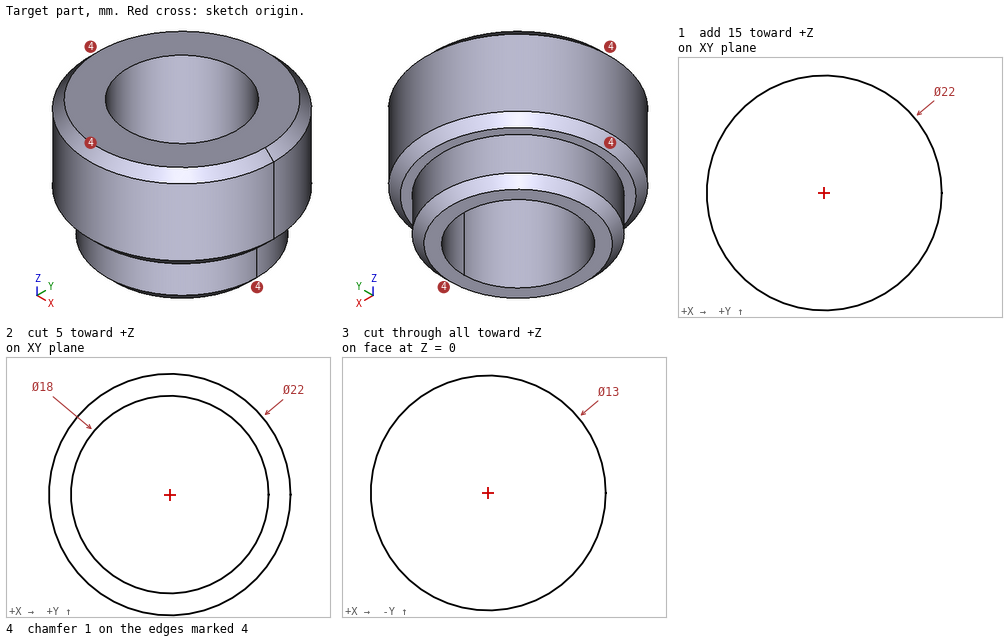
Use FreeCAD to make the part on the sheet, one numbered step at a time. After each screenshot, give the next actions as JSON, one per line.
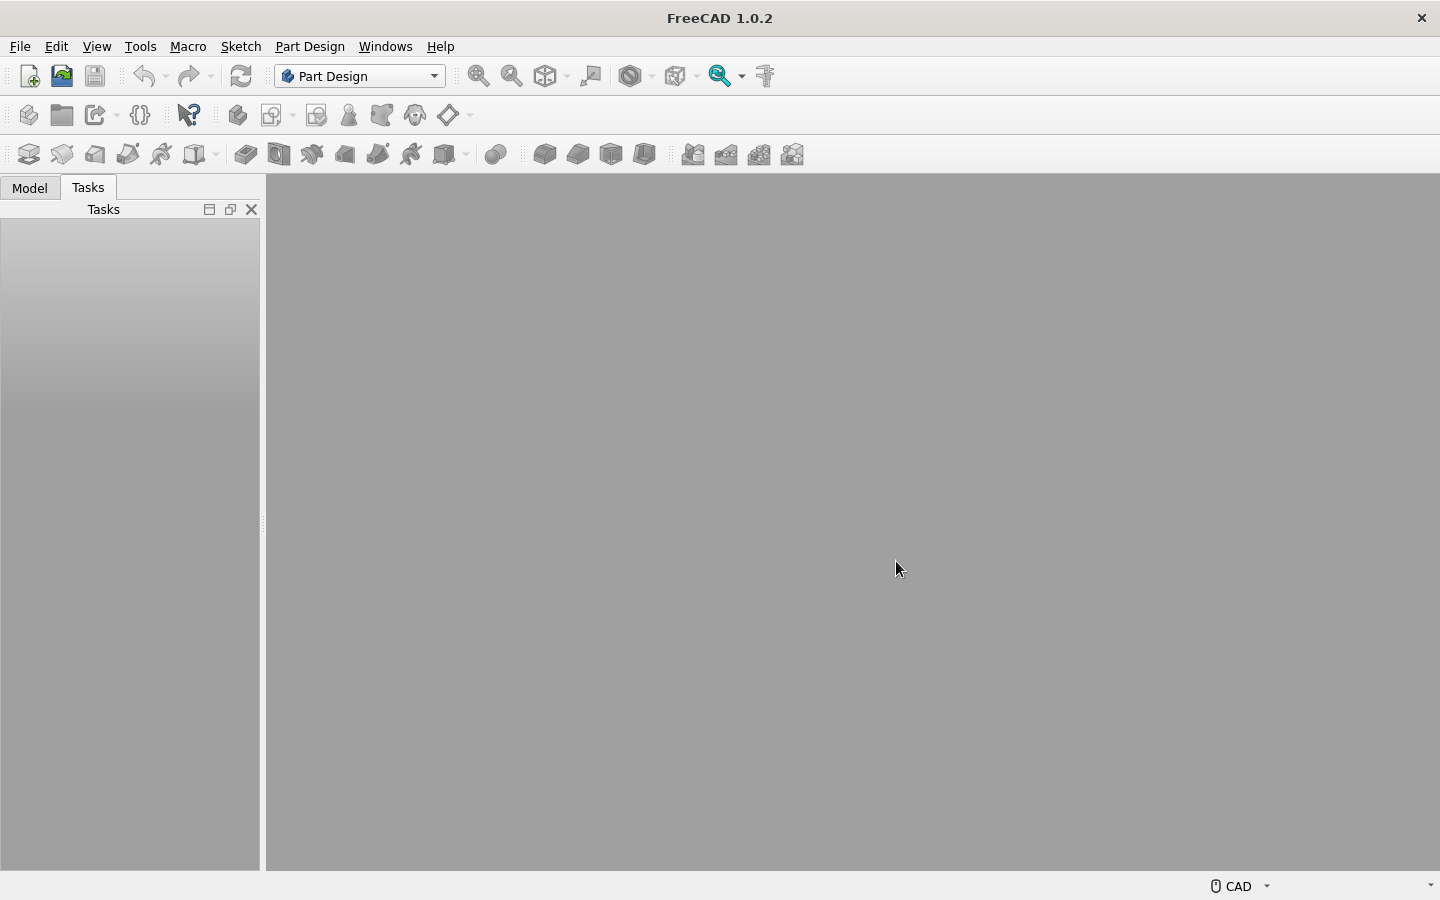
{"action": "key", "text": "ctrl+n"}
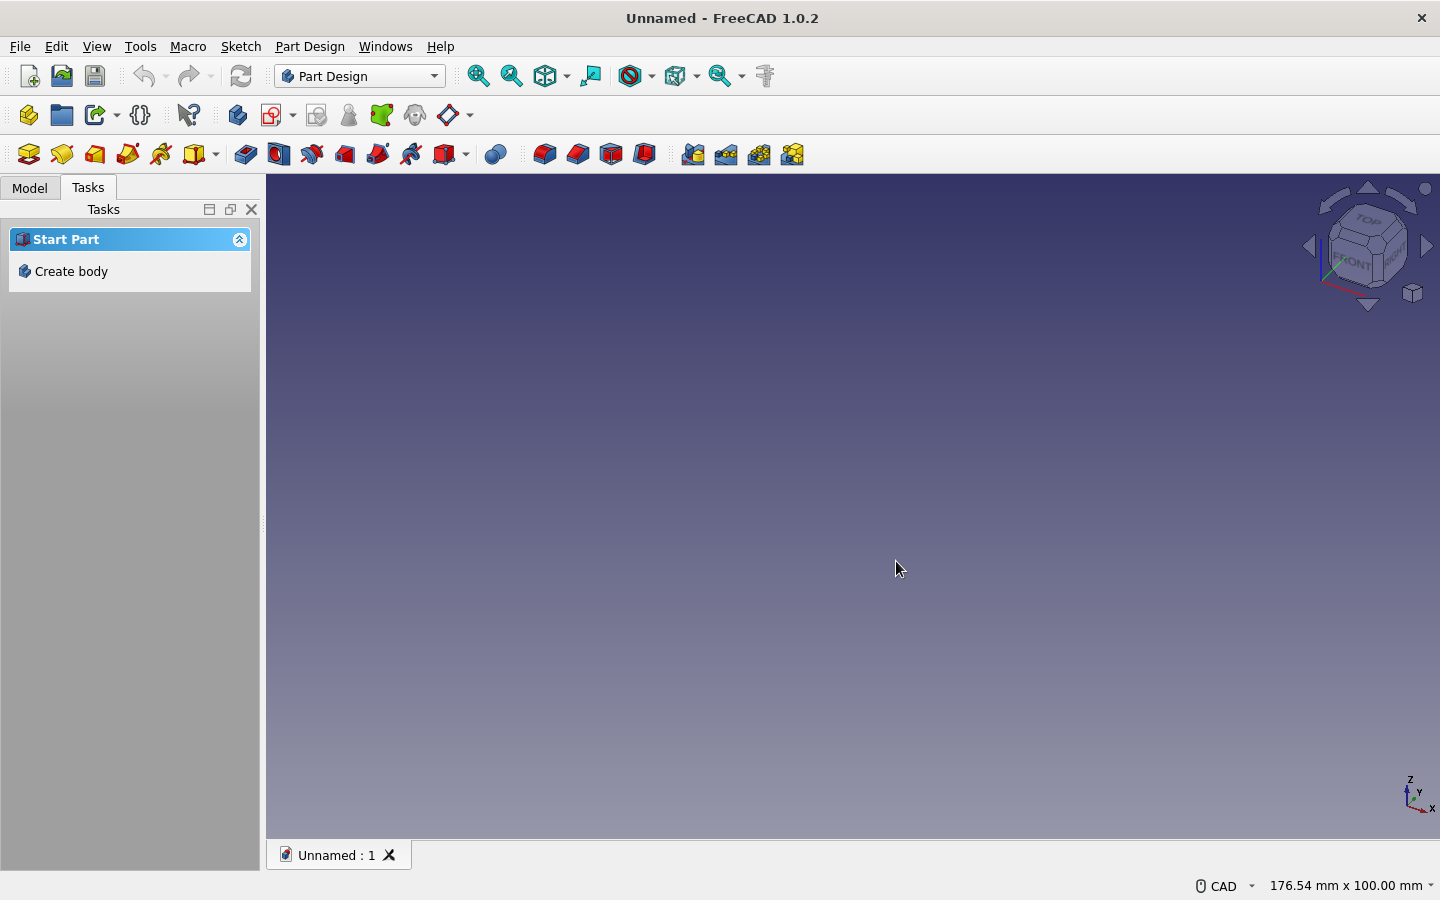
{"action": "left_click", "coordinate": [270, 116]}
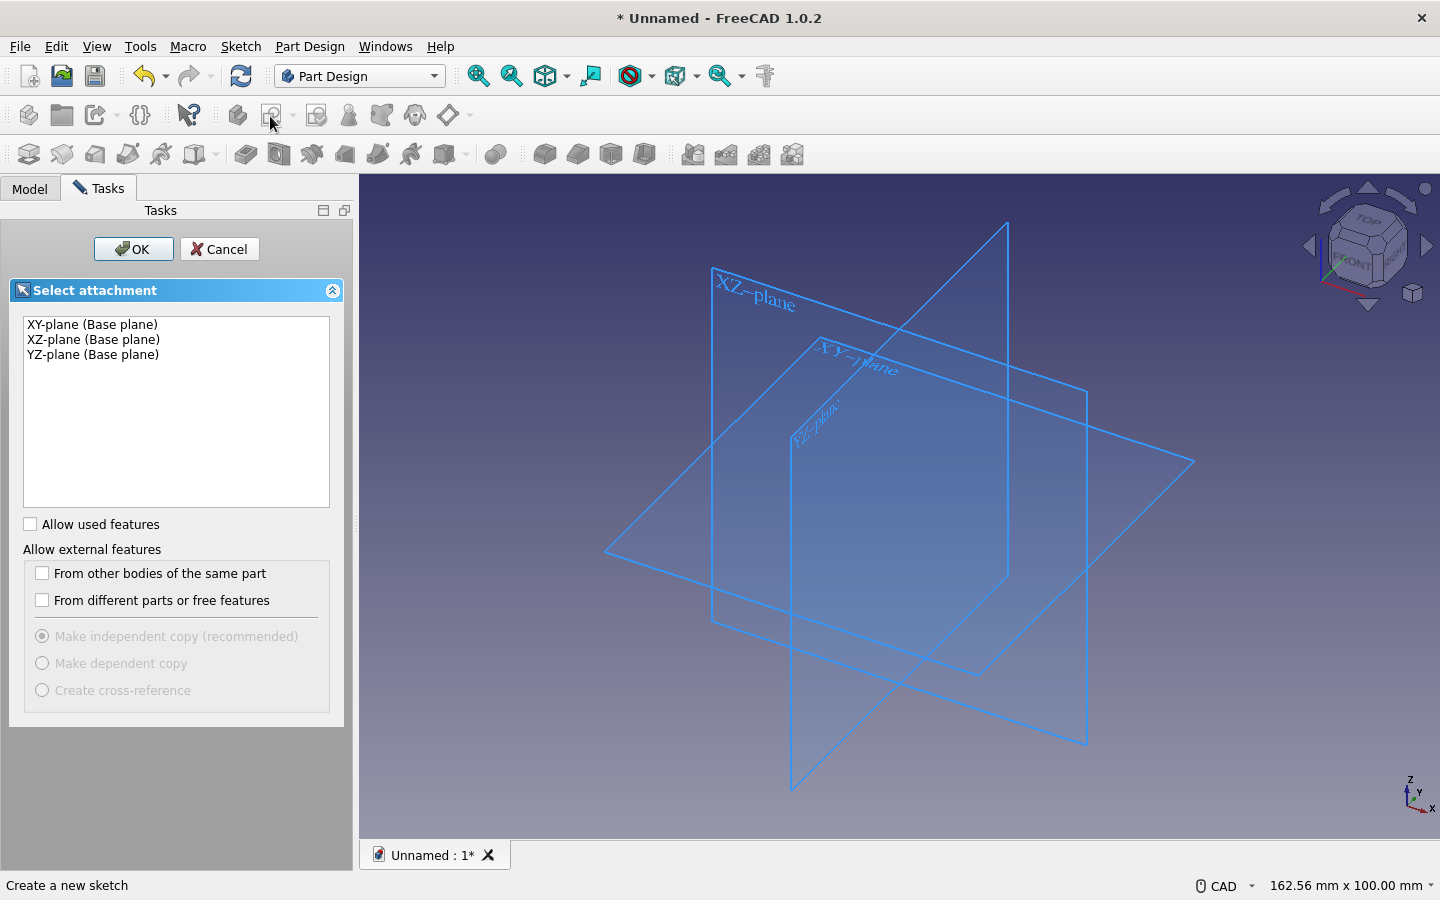
{"action": "left_click", "coordinate": [84, 324]}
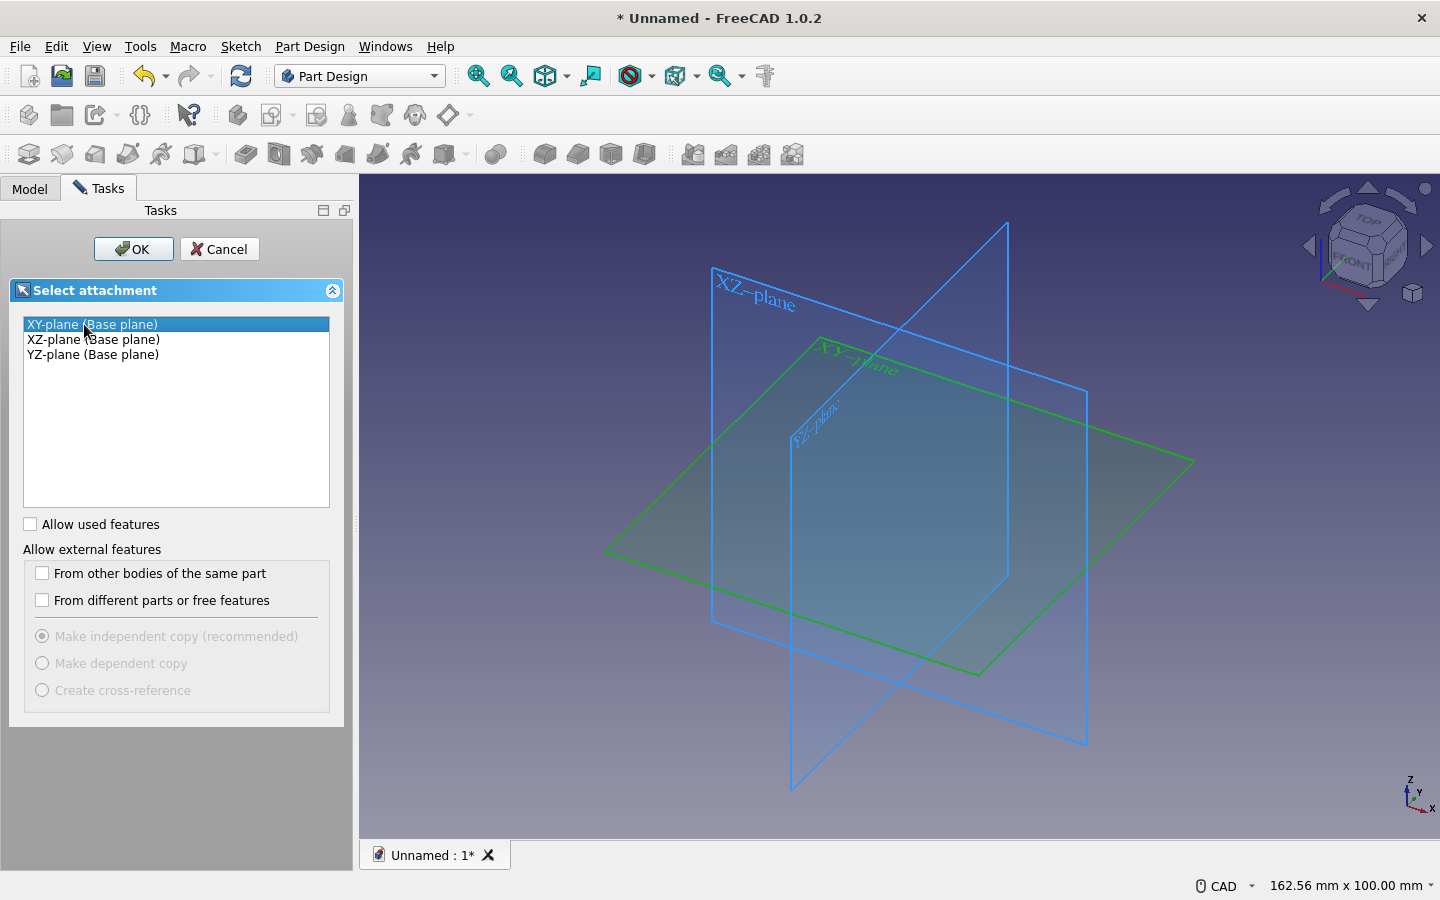
{"action": "left_click", "coordinate": [134, 249]}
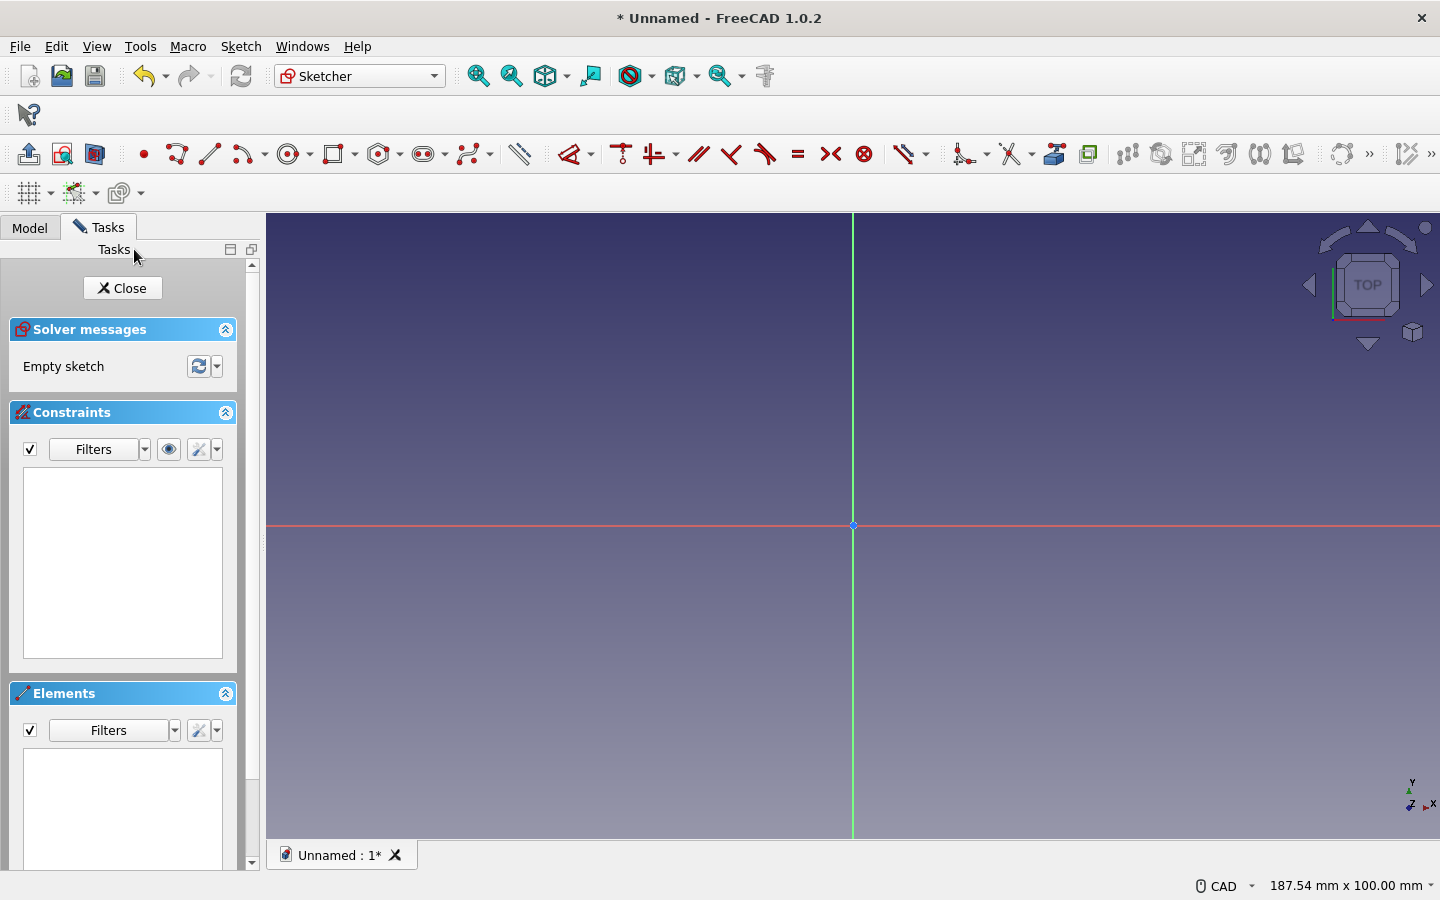
{"action": "scroll", "coordinate": [893, 526], "scroll_direction": "up", "scroll_amount": 5}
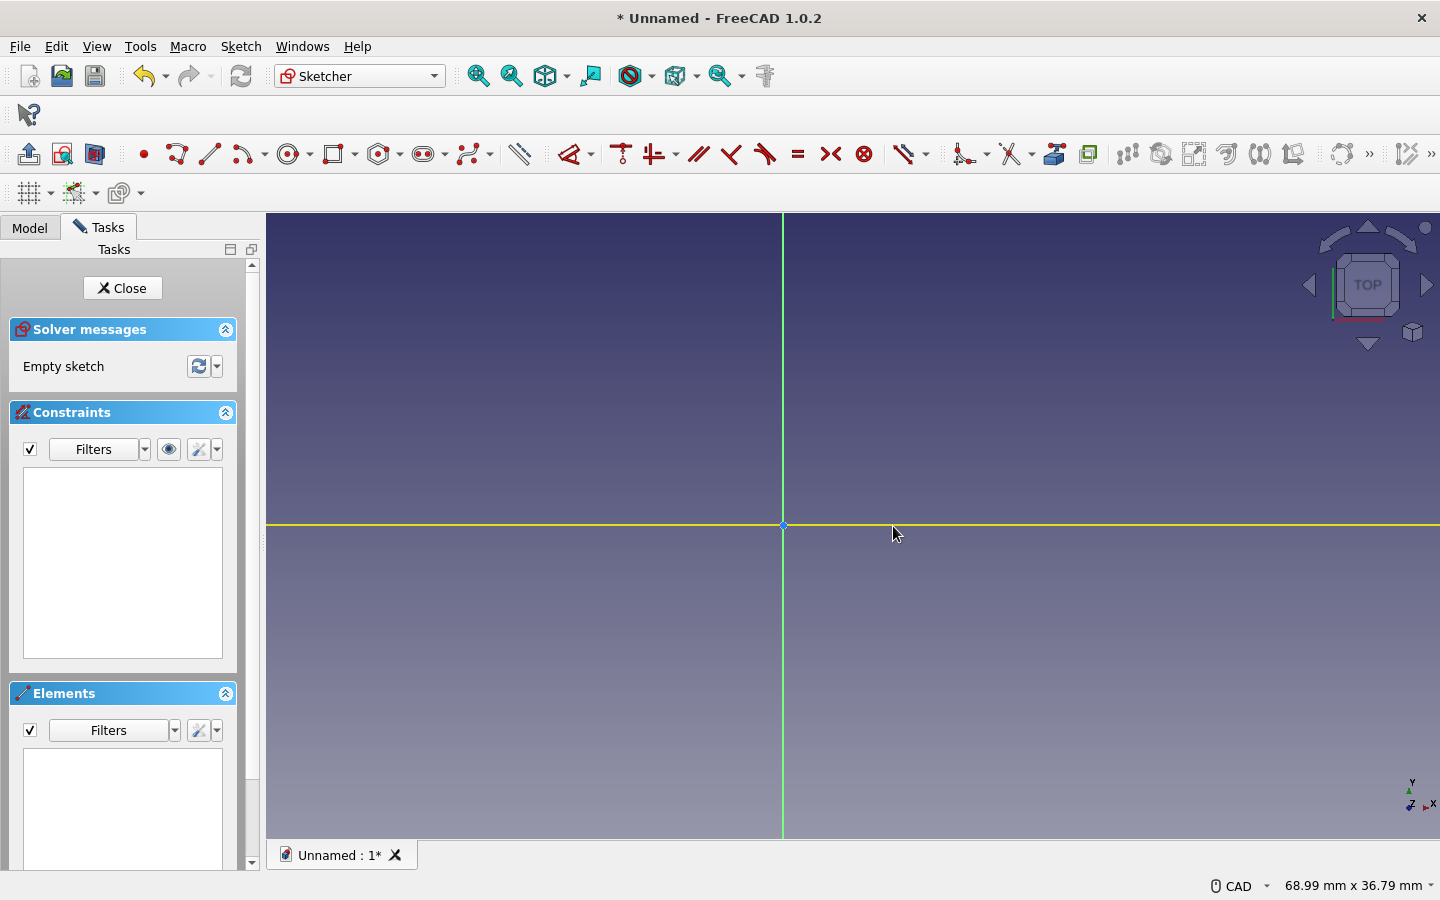
{"action": "left_click", "coordinate": [288, 154]}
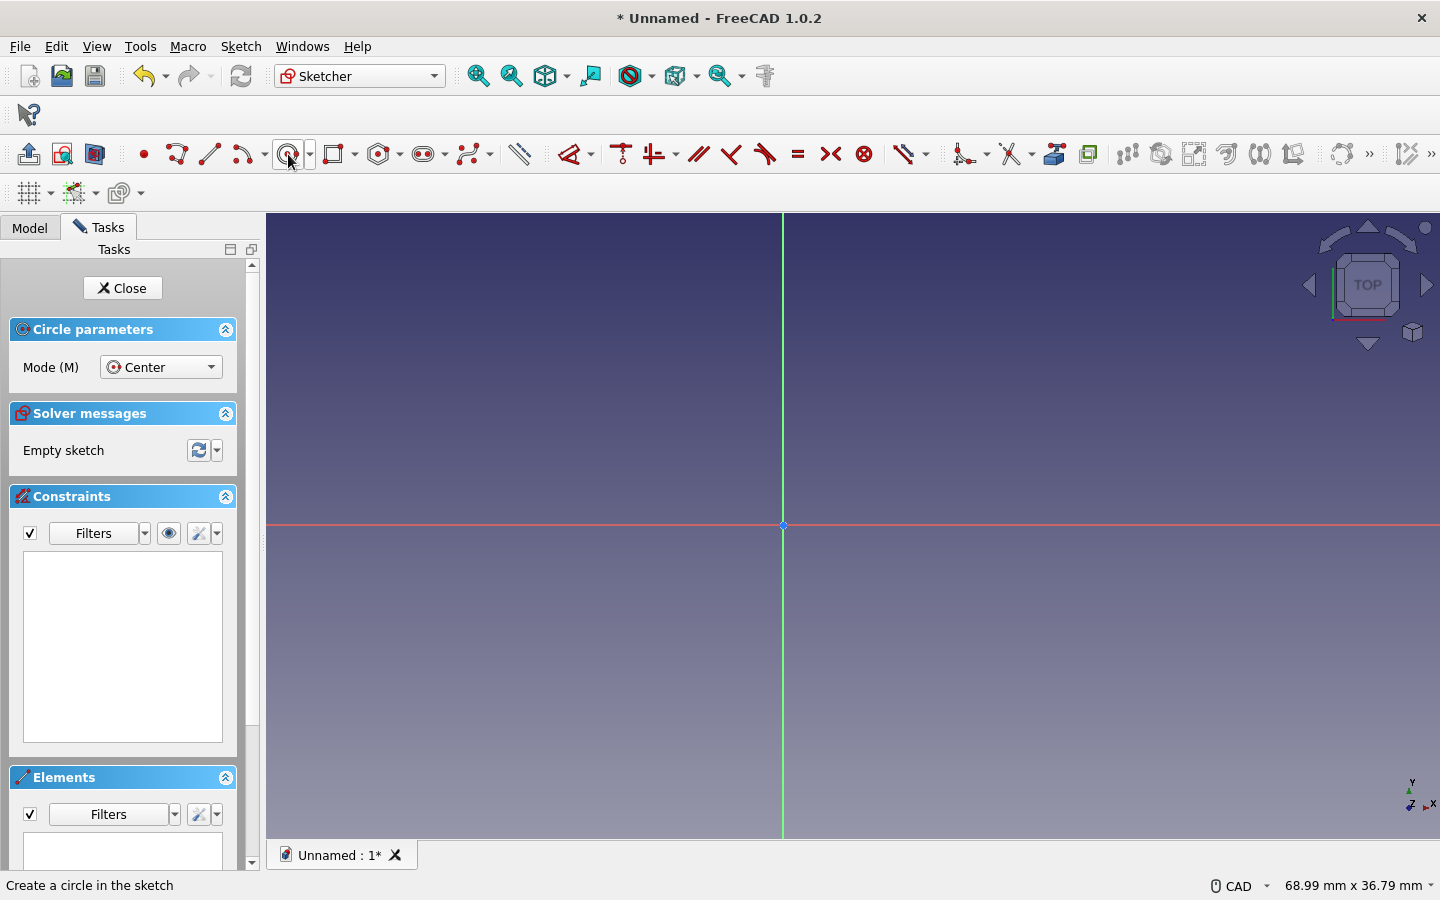
{"action": "left_click", "coordinate": [783, 525]}
{"action": "mouse_move", "coordinate": [916, 393]}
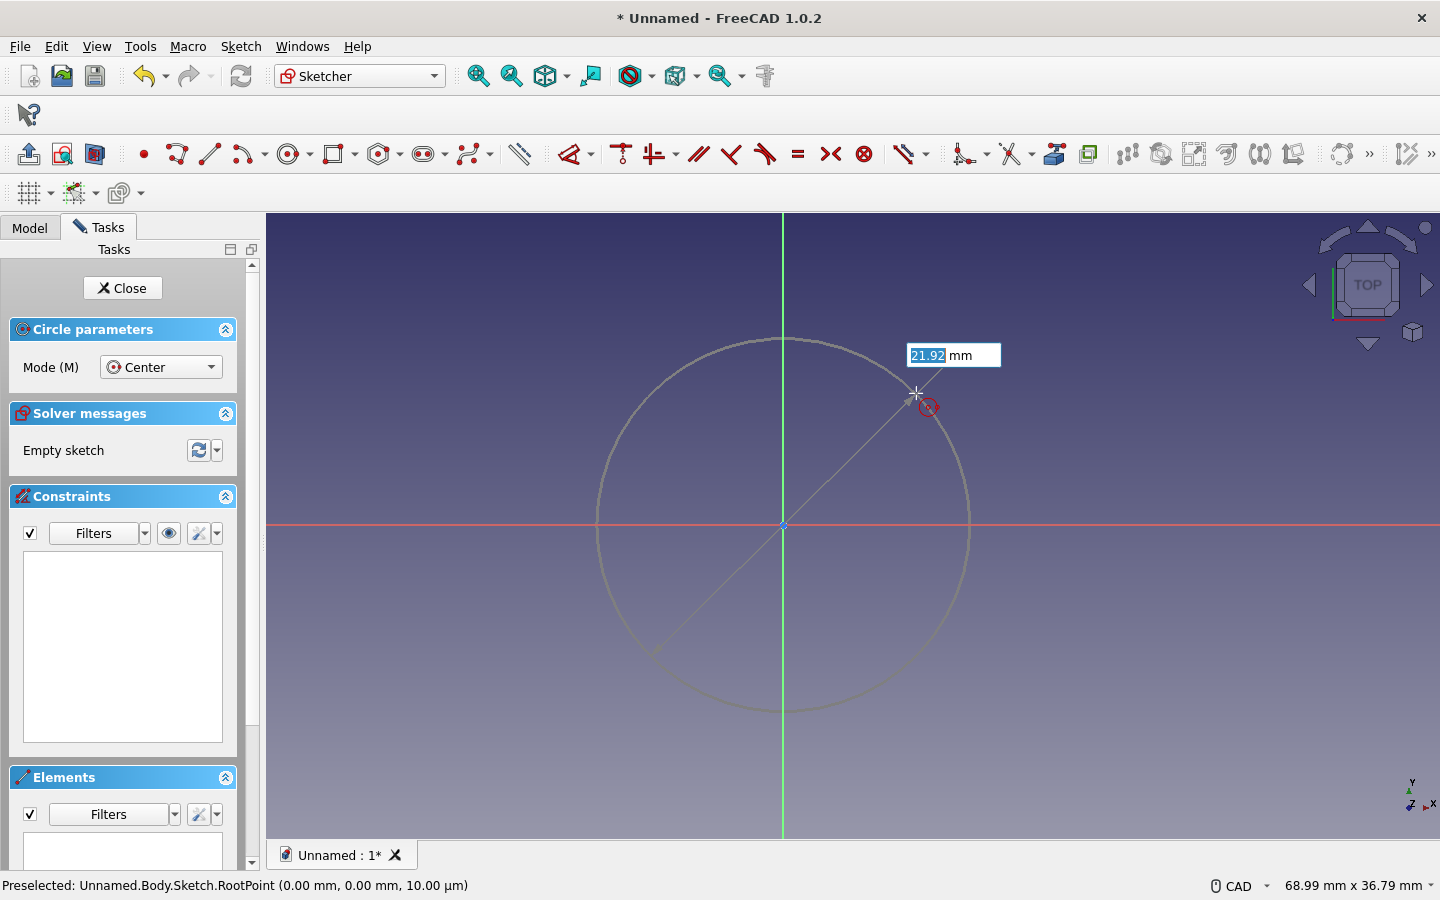
{"action": "type", "text": "22"}
{"action": "key", "text": "Return"}
{"action": "key", "text": "Escape"}